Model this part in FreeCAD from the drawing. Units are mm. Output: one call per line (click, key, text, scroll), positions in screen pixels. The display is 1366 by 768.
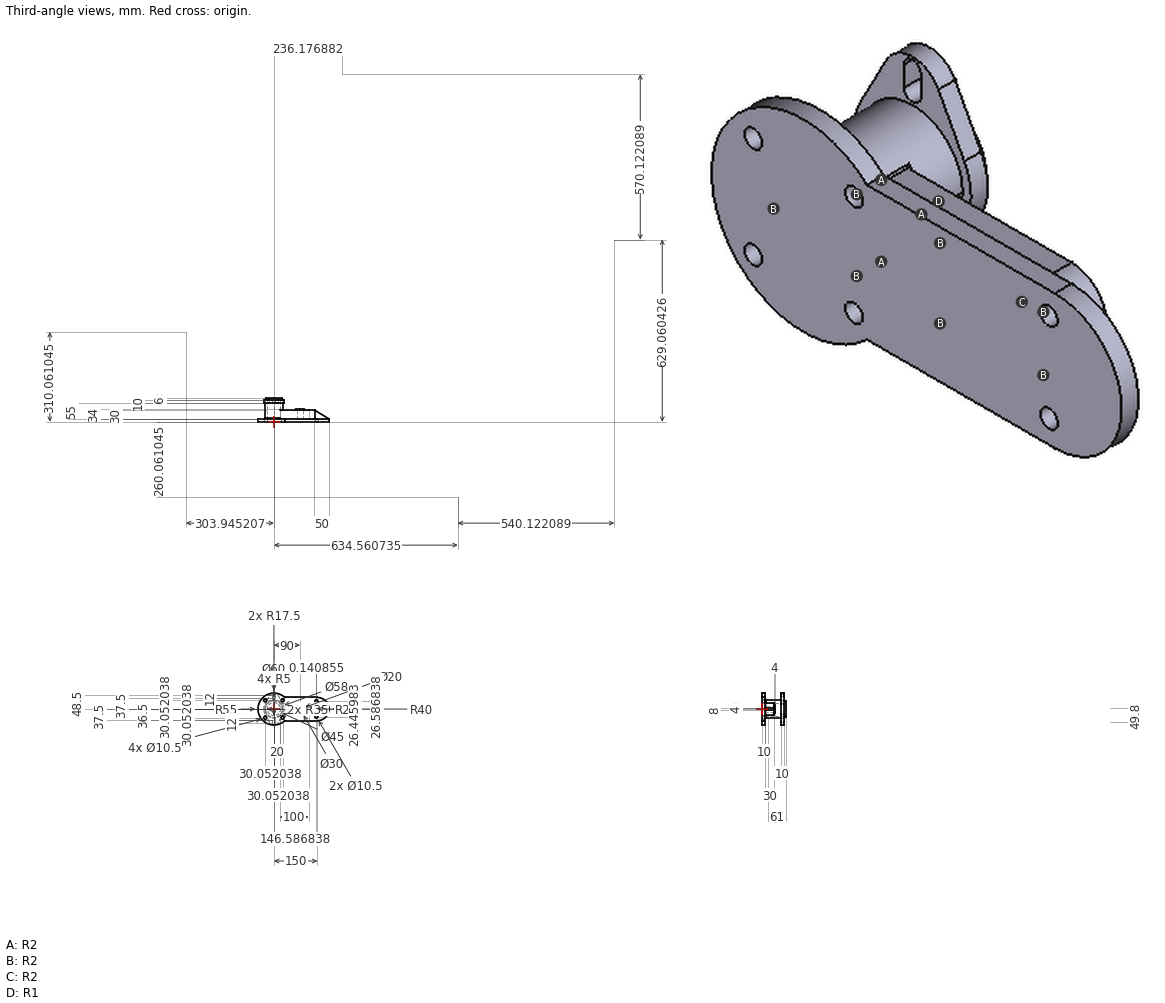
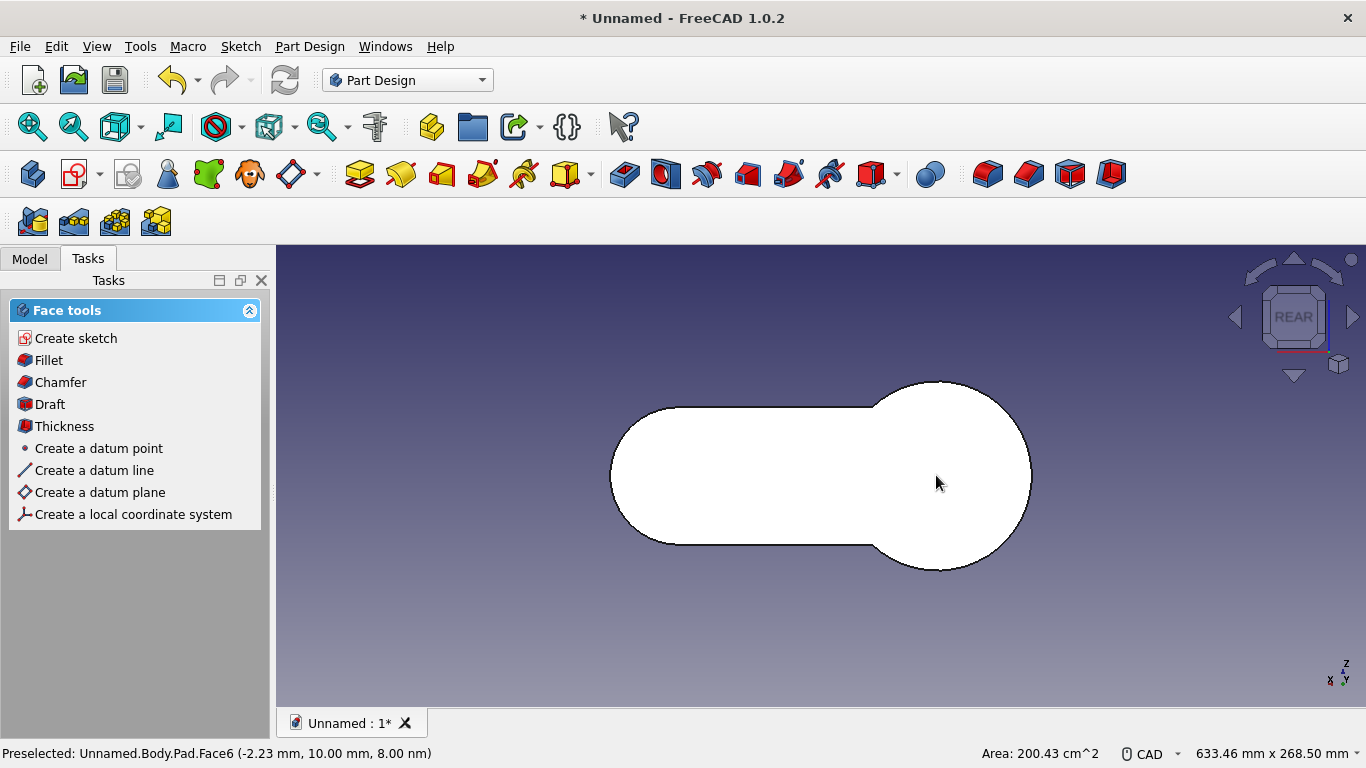
click(74, 174)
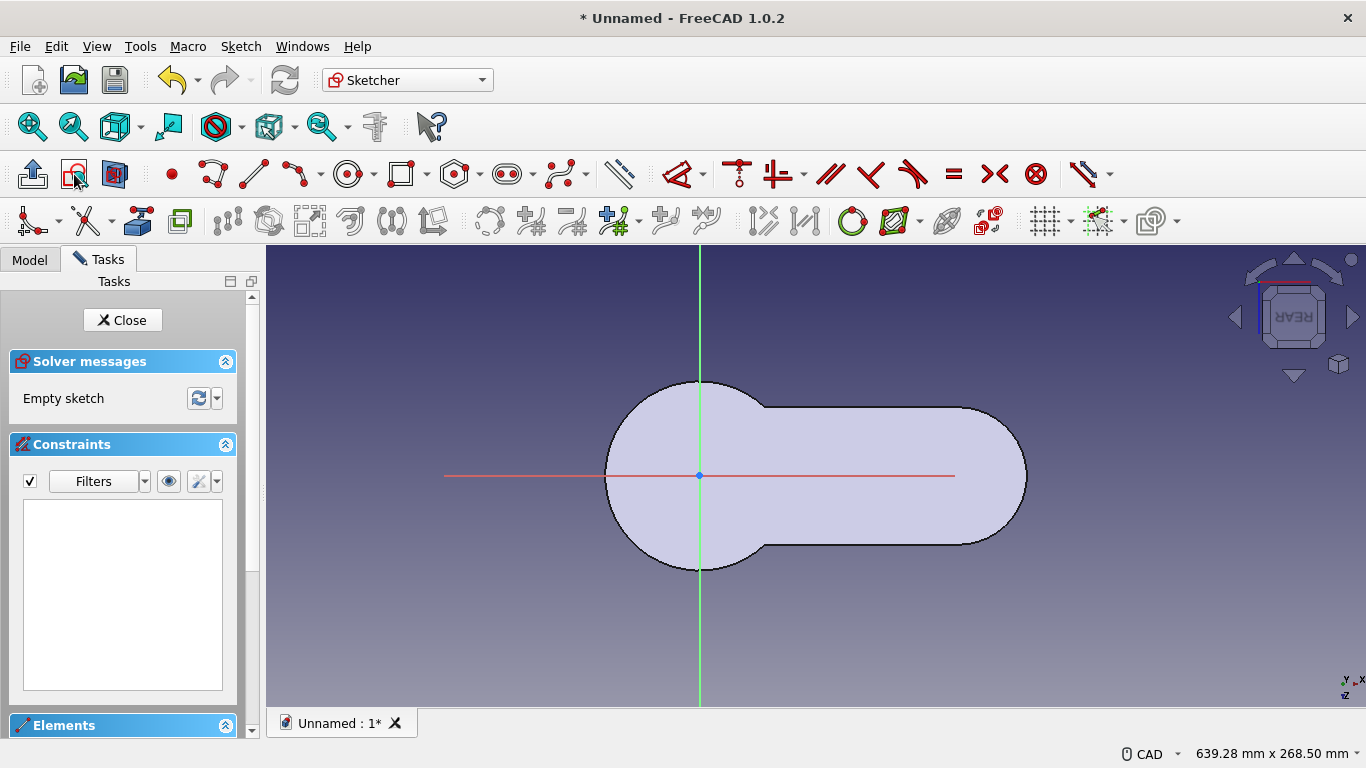
scroll(672, 476, up, 5)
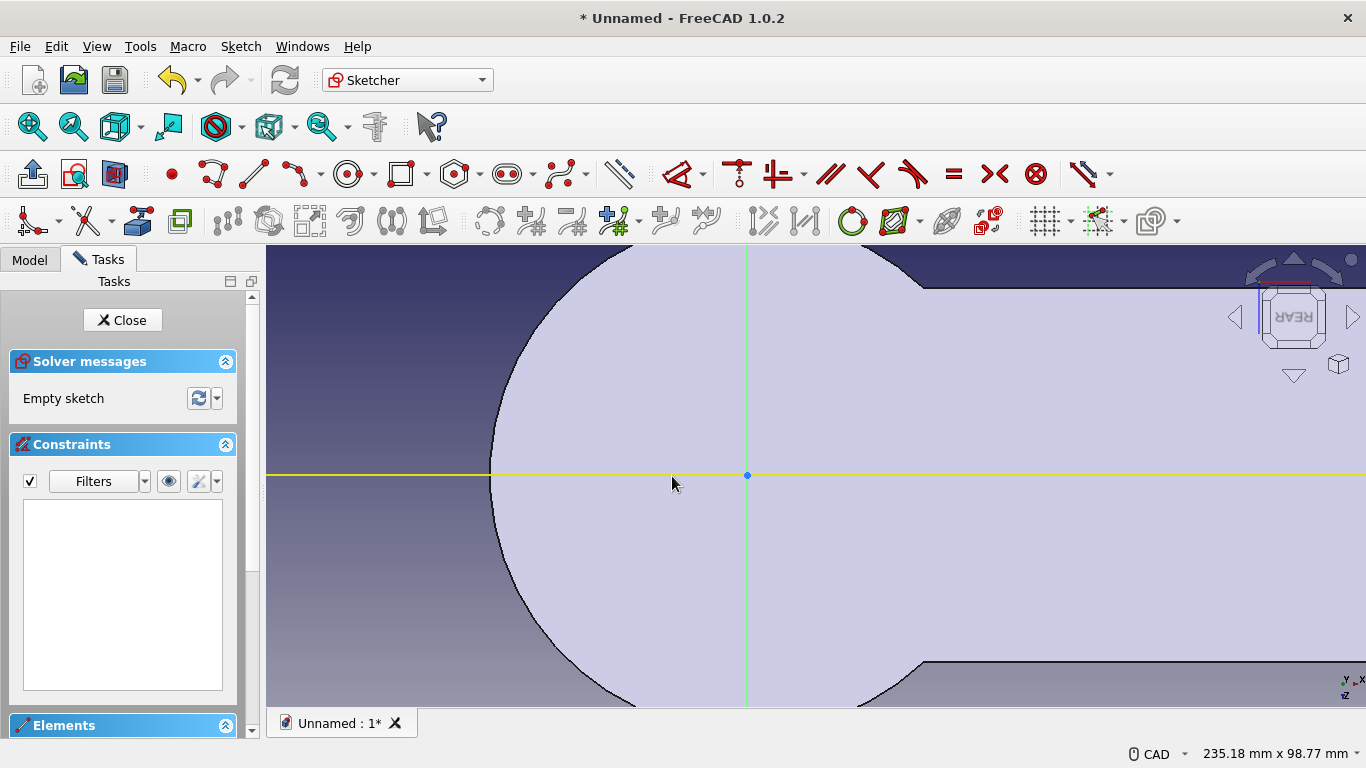
key(g)
key(c)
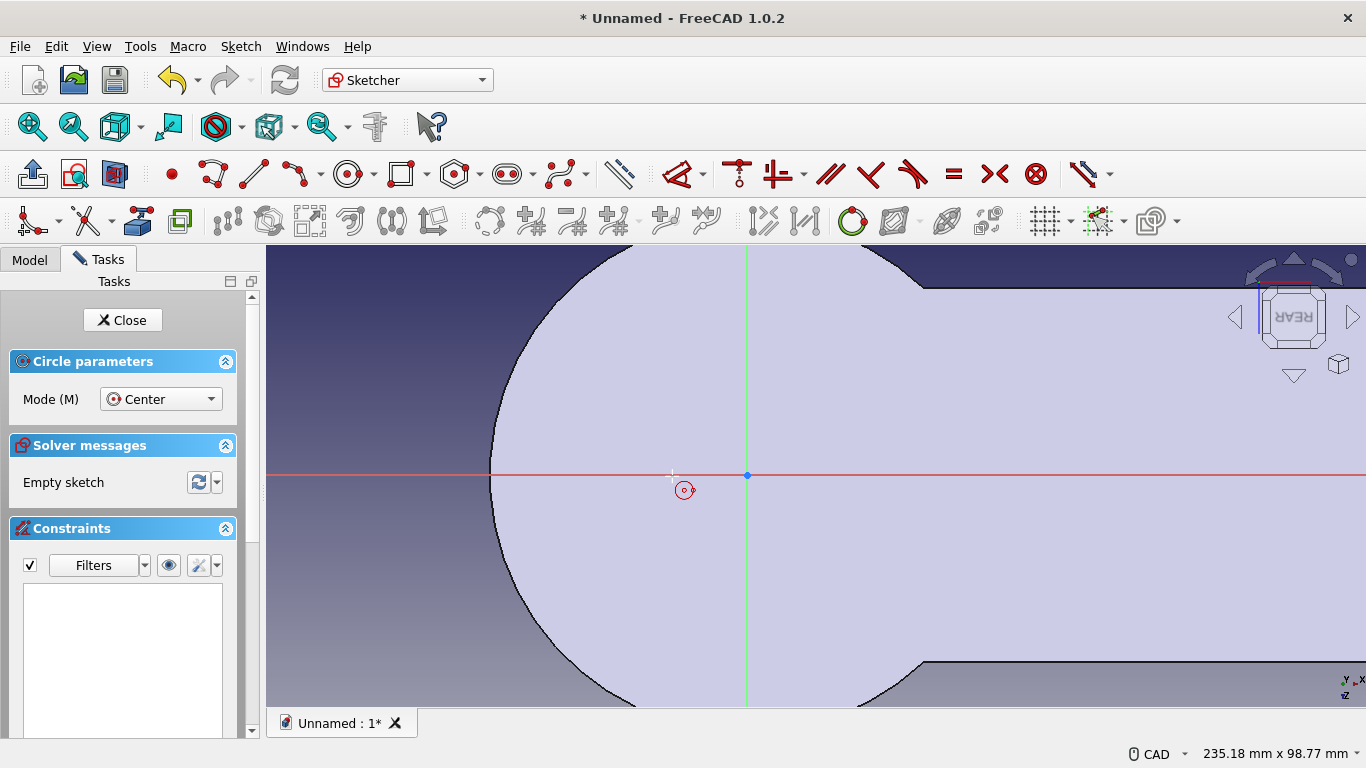
click(747, 475)
click(846, 376)
key(Escape)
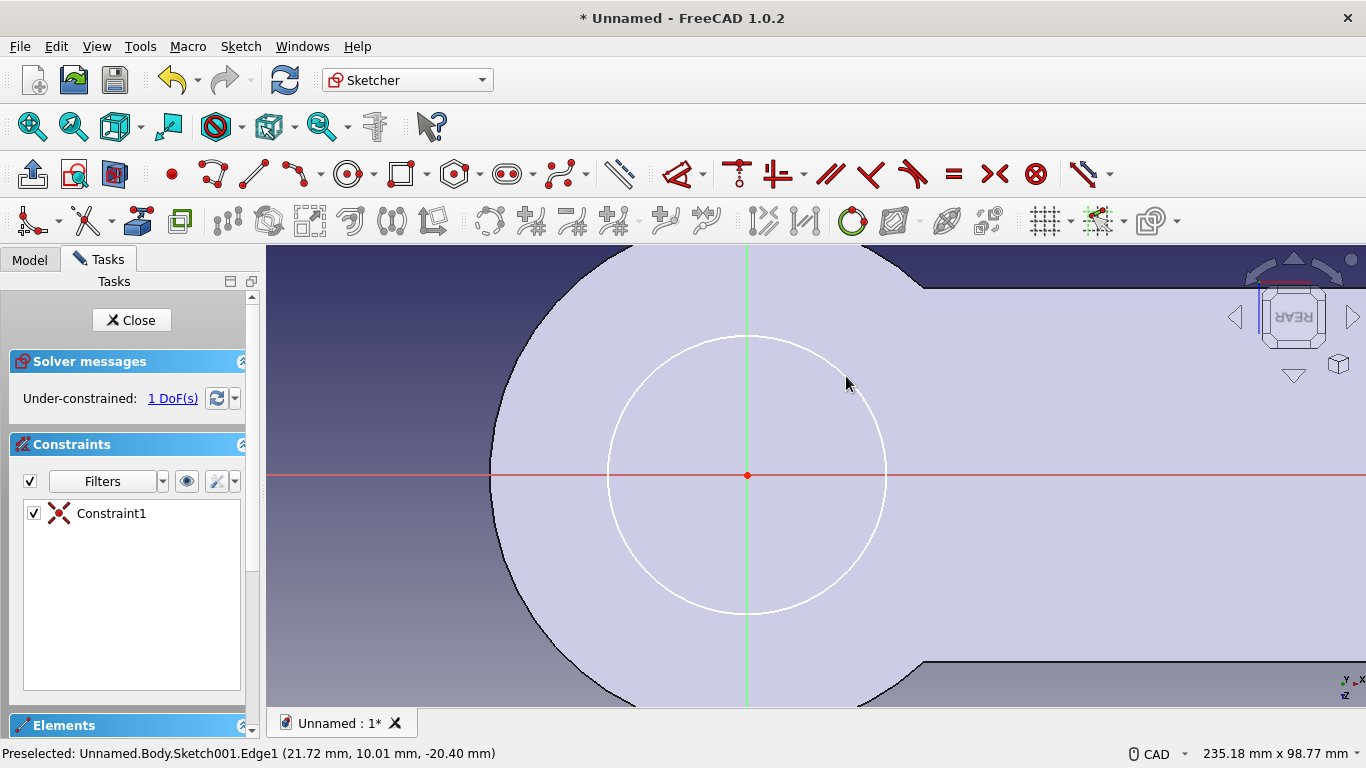
key(d)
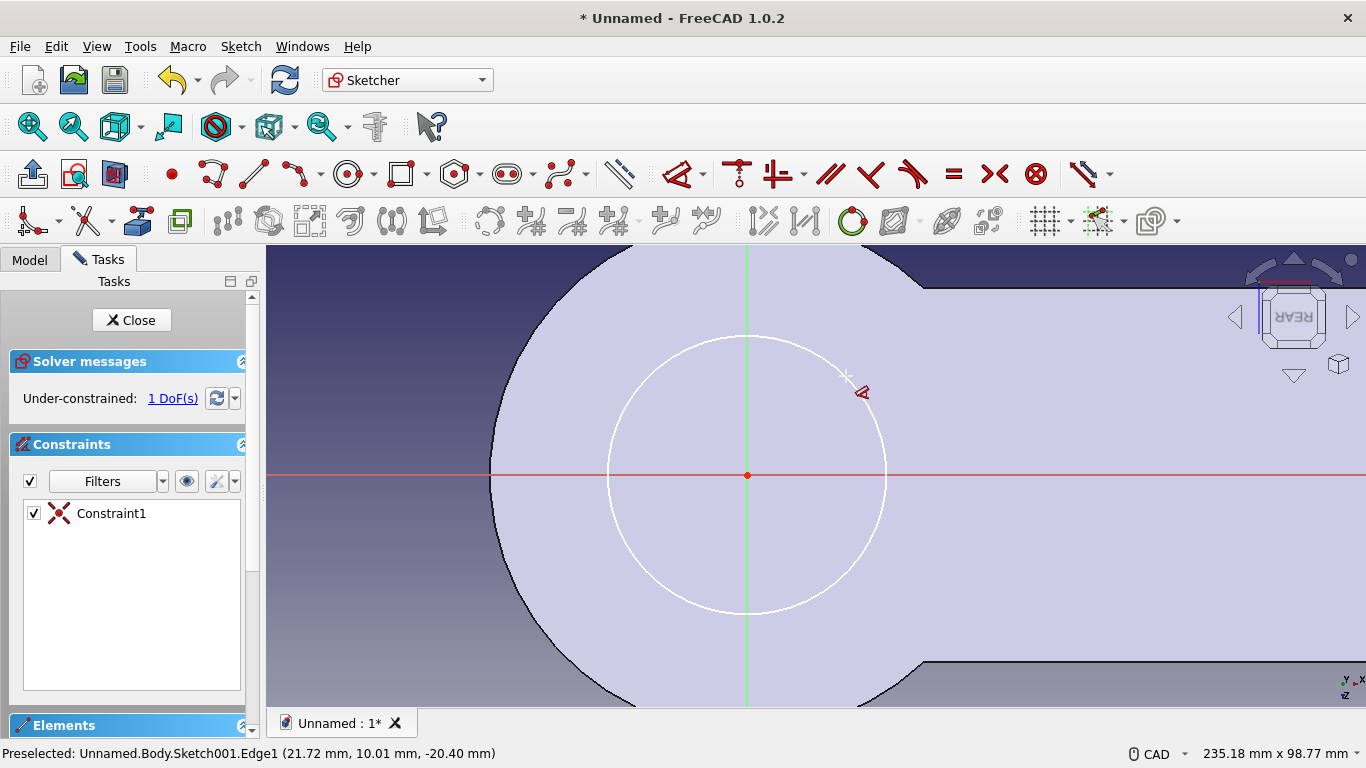
click(845, 376)
click(867, 353)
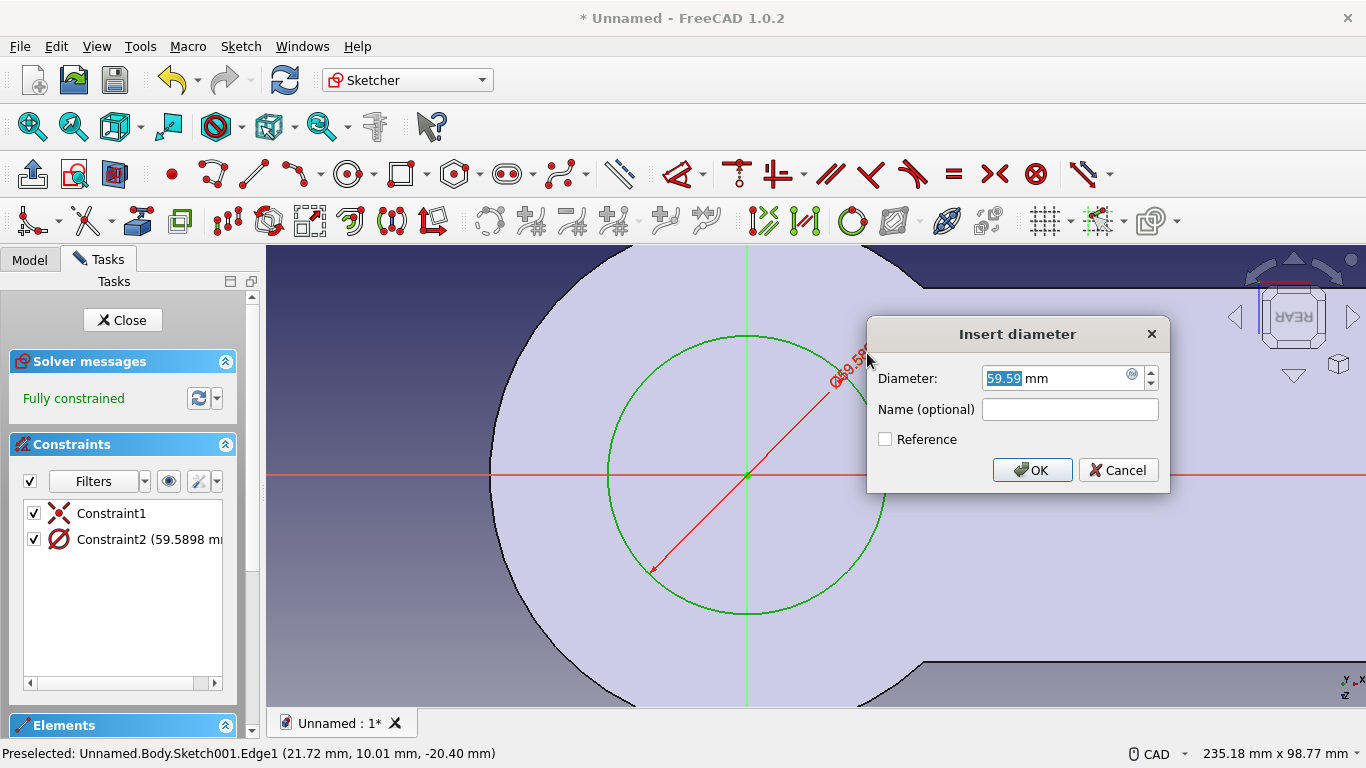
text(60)
key(Return)
key(Escape)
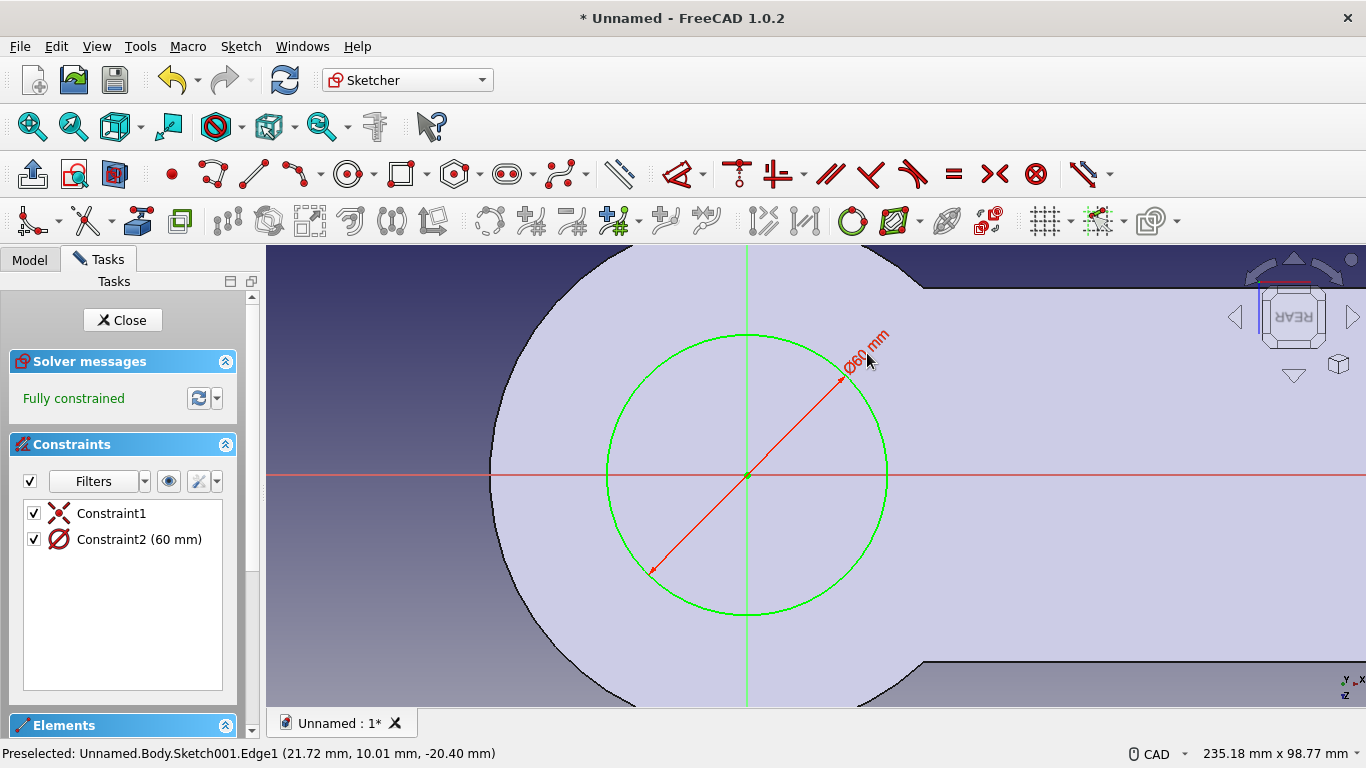
click(123, 320)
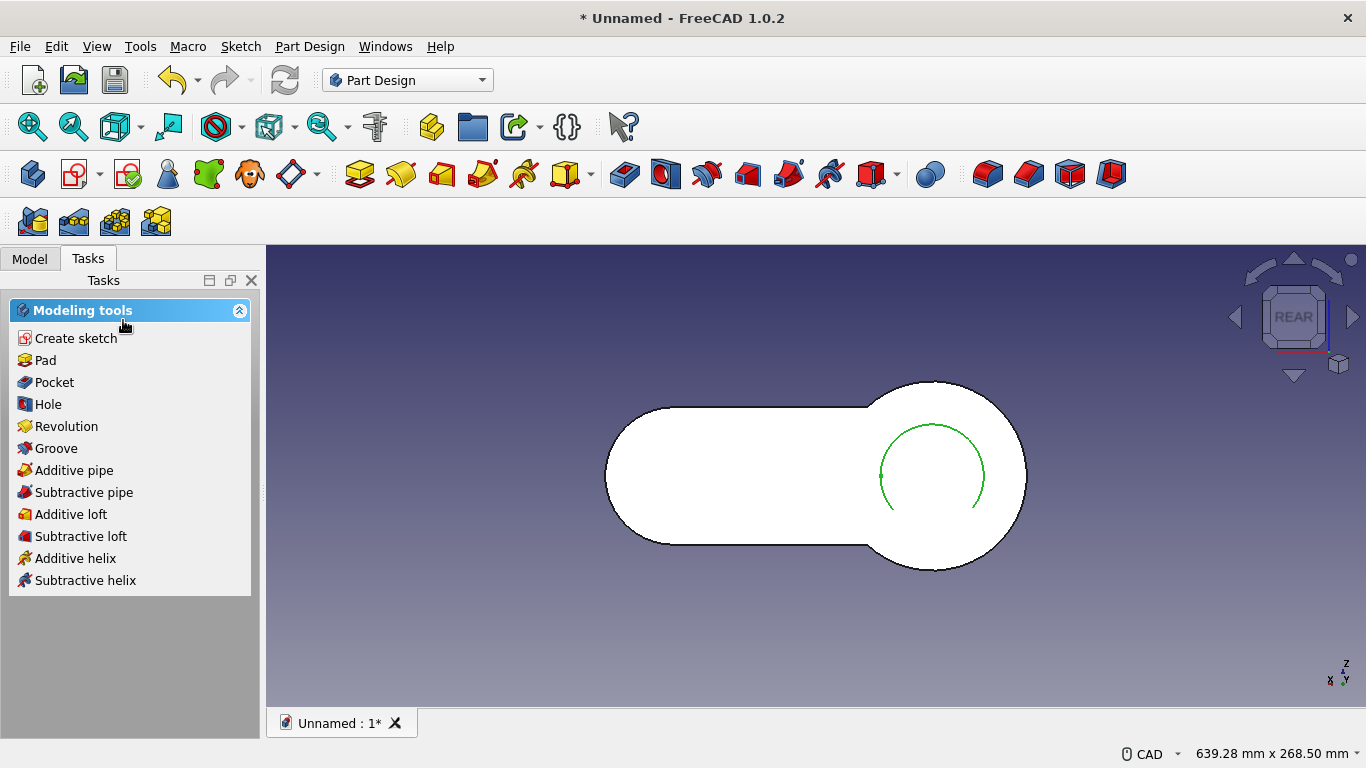
click(360, 174)